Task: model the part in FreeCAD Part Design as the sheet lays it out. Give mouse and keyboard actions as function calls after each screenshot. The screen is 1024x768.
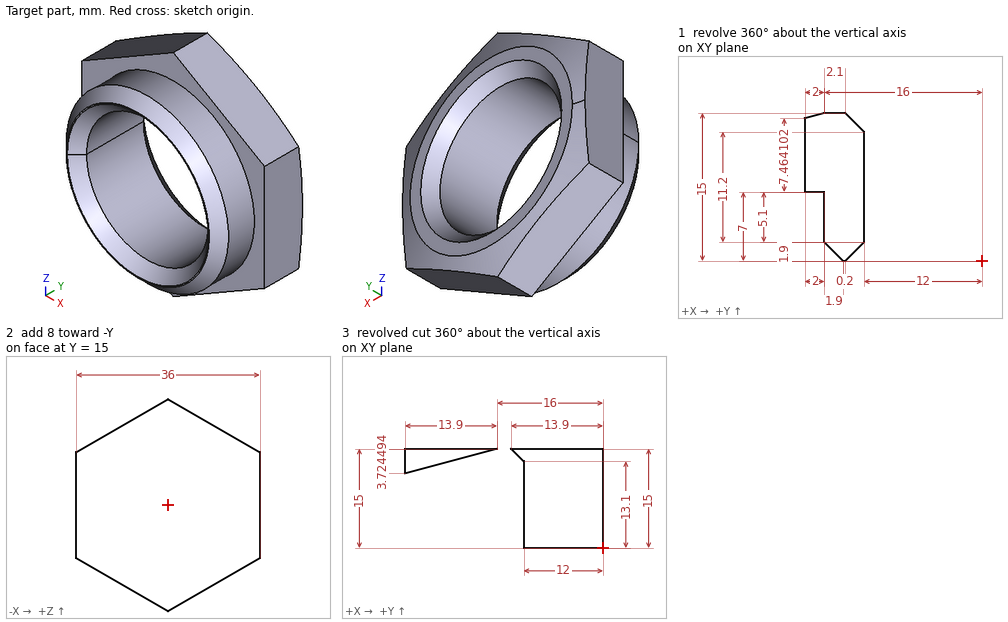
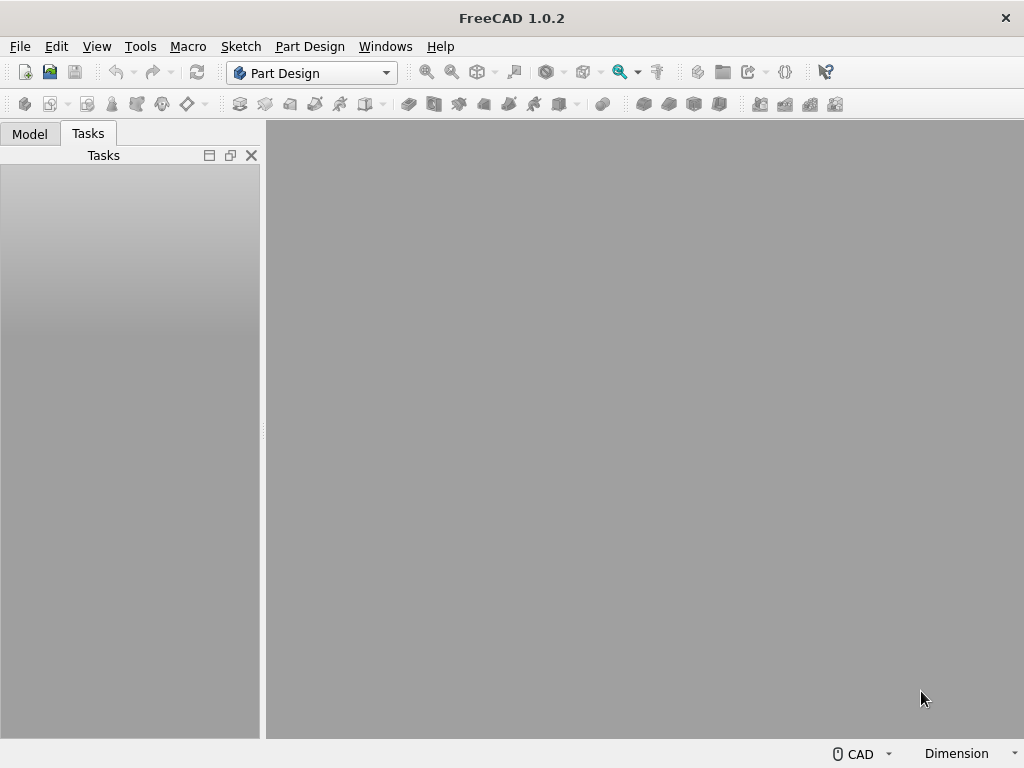
click(25, 72)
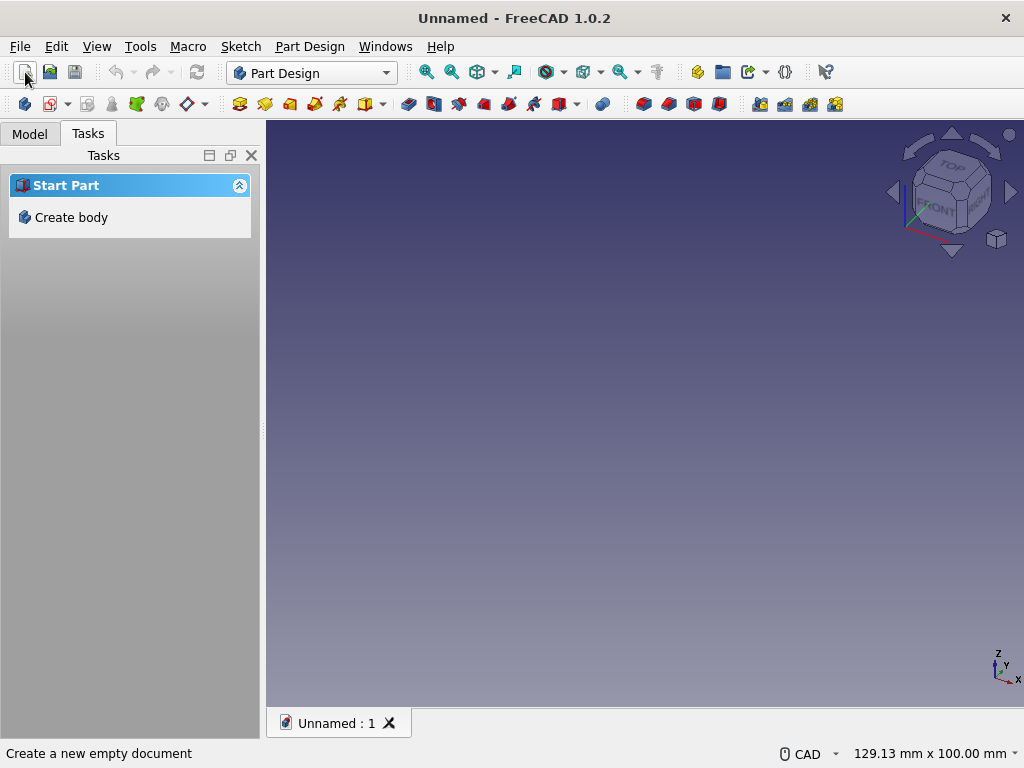
click(50, 104)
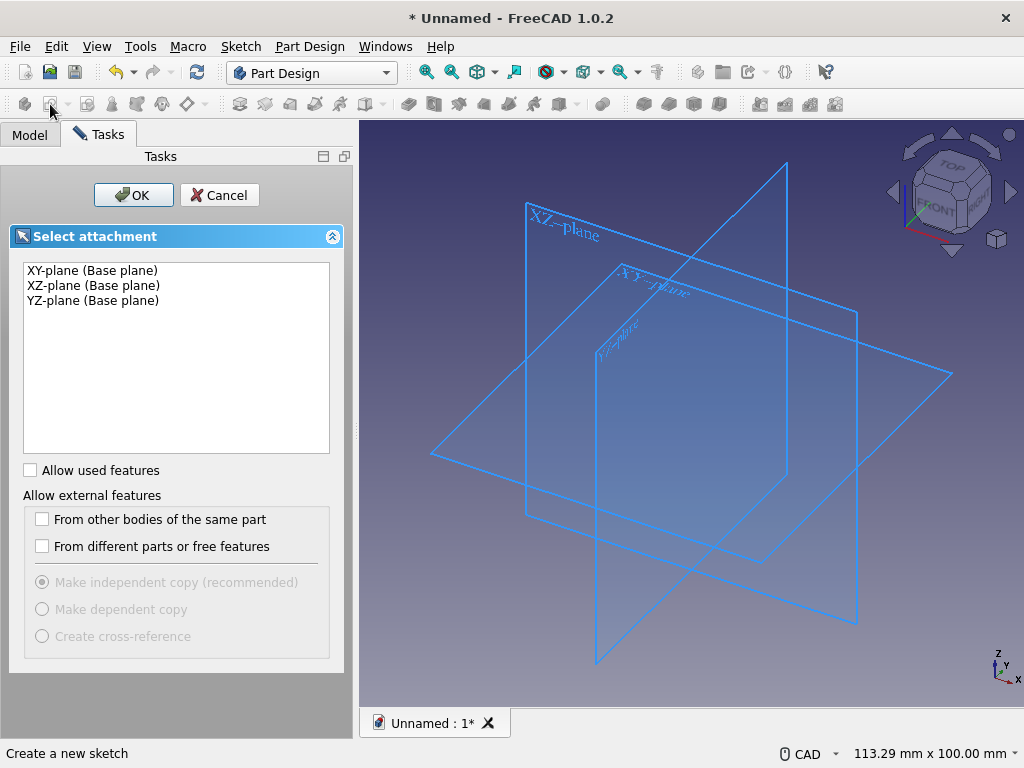
click(84, 270)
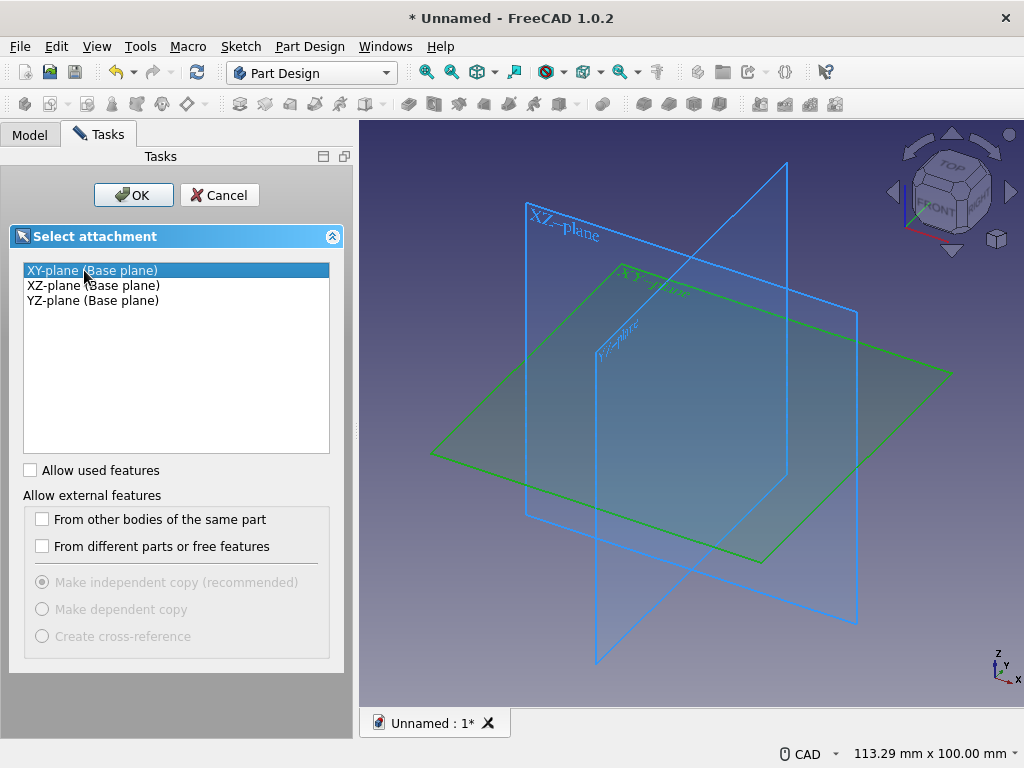
click(134, 195)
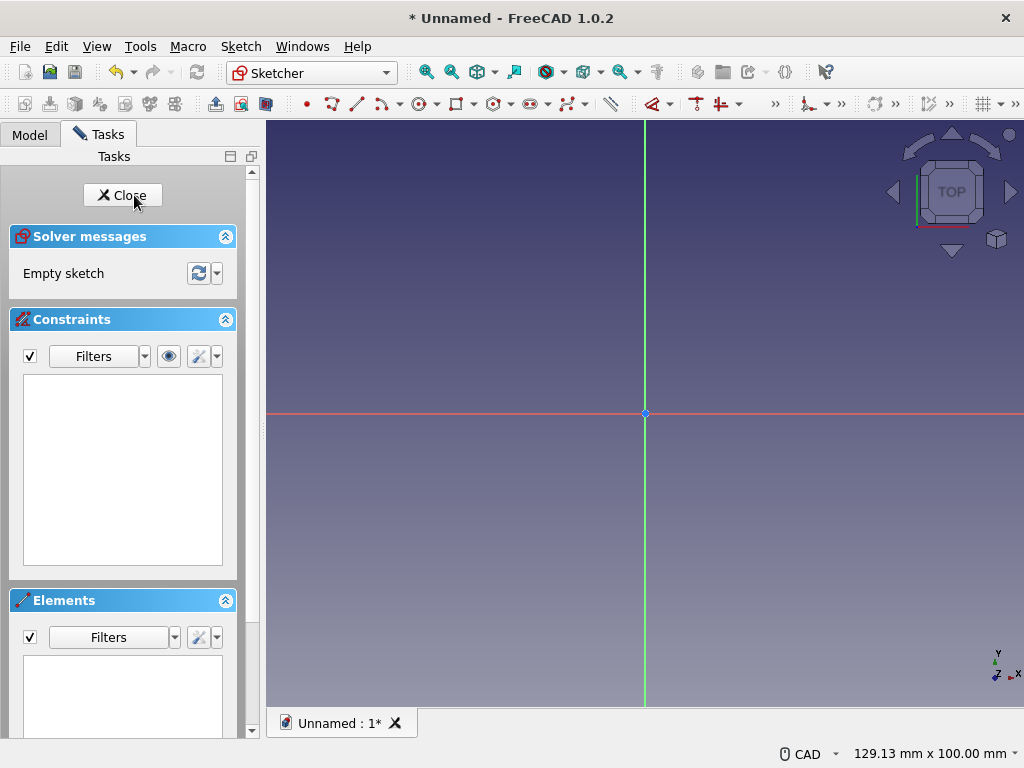
scroll(597, 355, up, 7)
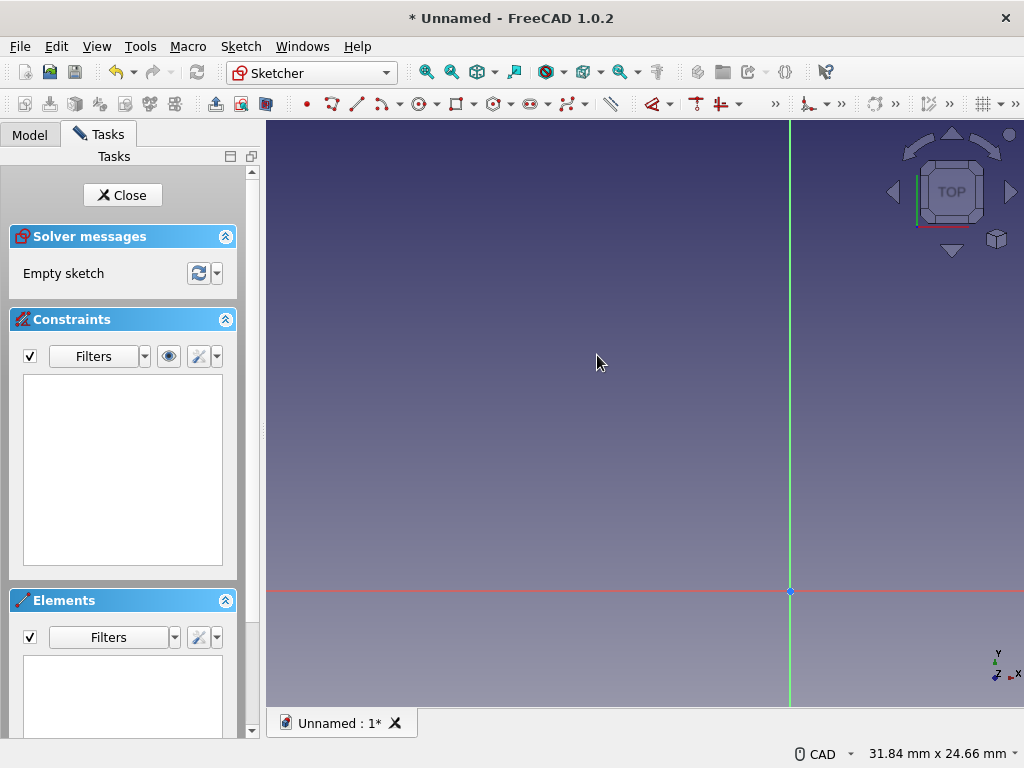
key(g)
key(m)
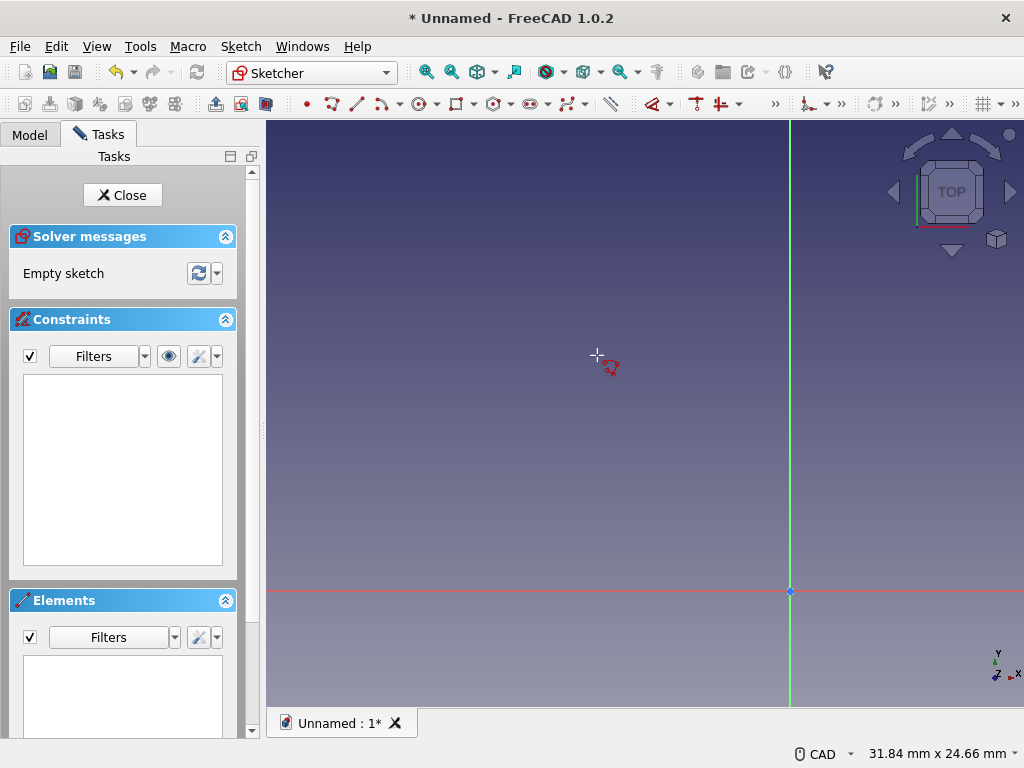
click(505, 546)
click(505, 279)
click(459, 234)
click(409, 234)
click(362, 247)
click(362, 424)
click(409, 424)
click(409, 546)
click(455, 591)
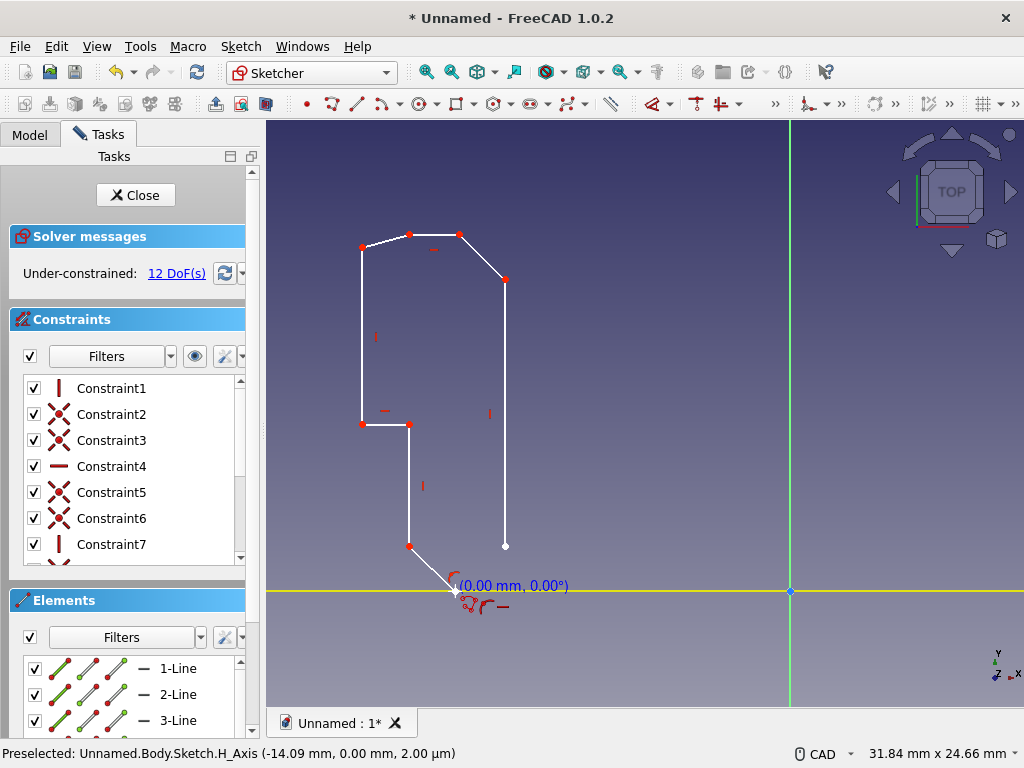
scroll(459, 591, up, 7)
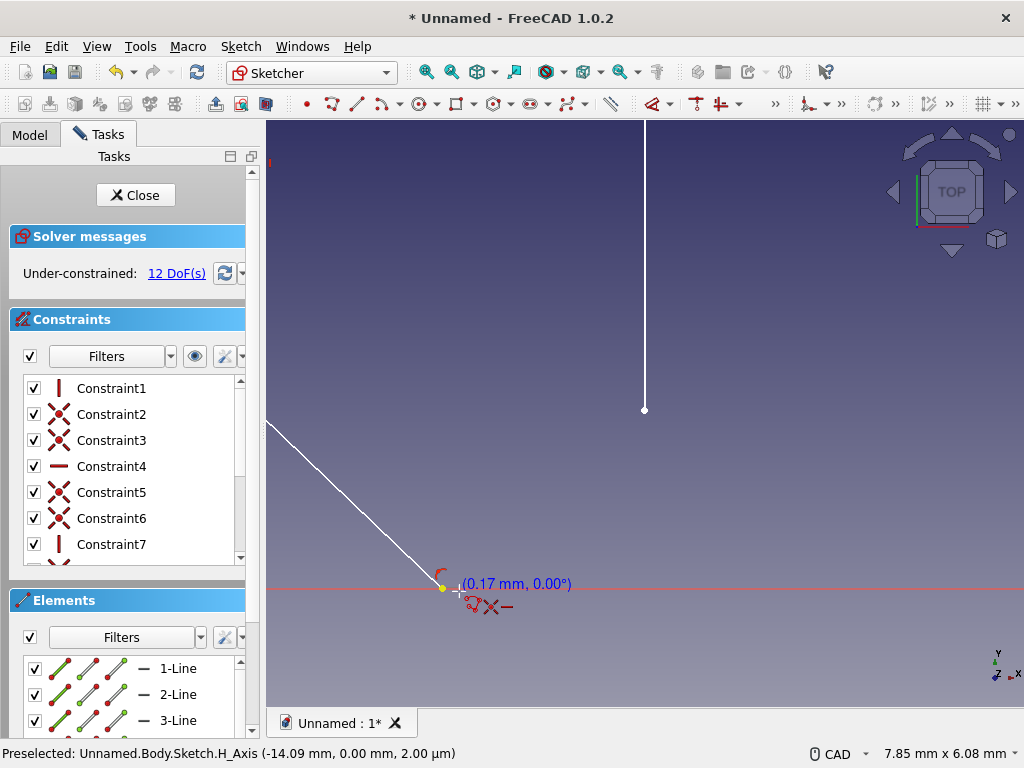
click(460, 580)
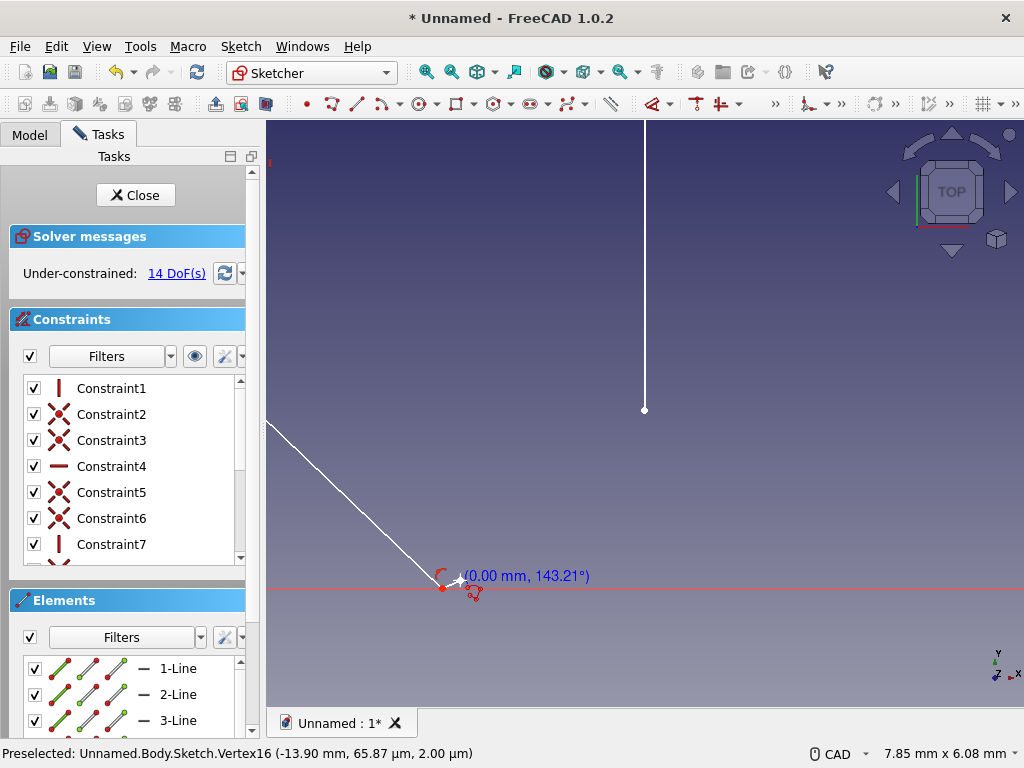
scroll(460, 593, down, 7)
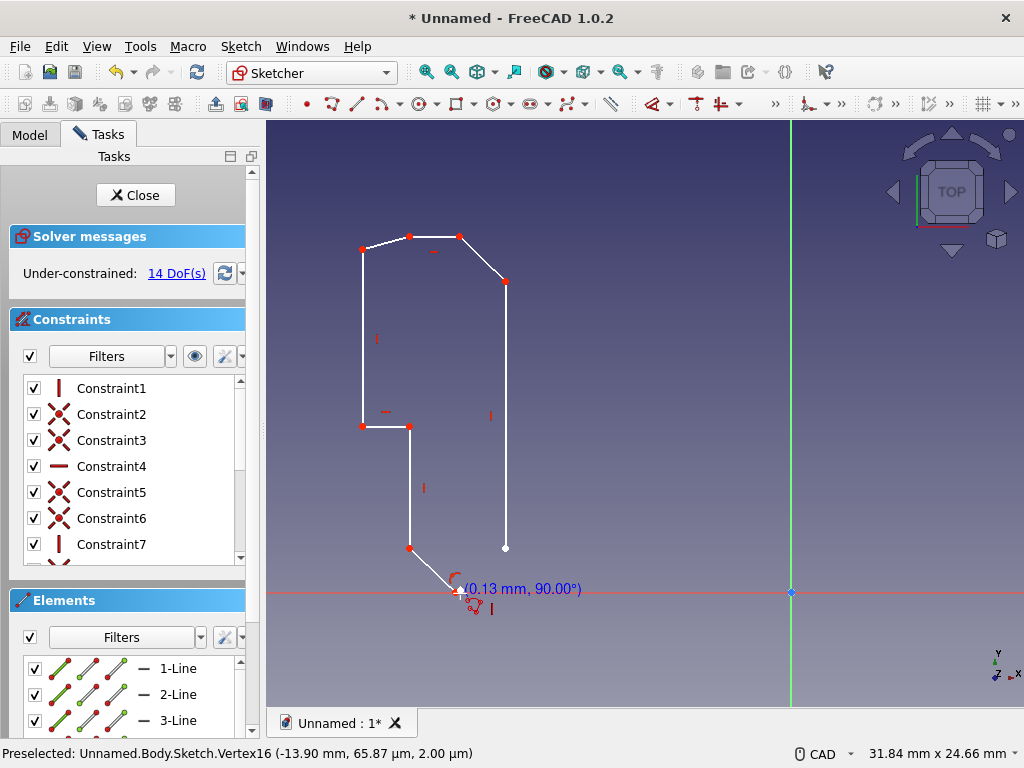
click(506, 549)
key(Escape)
key(Escape)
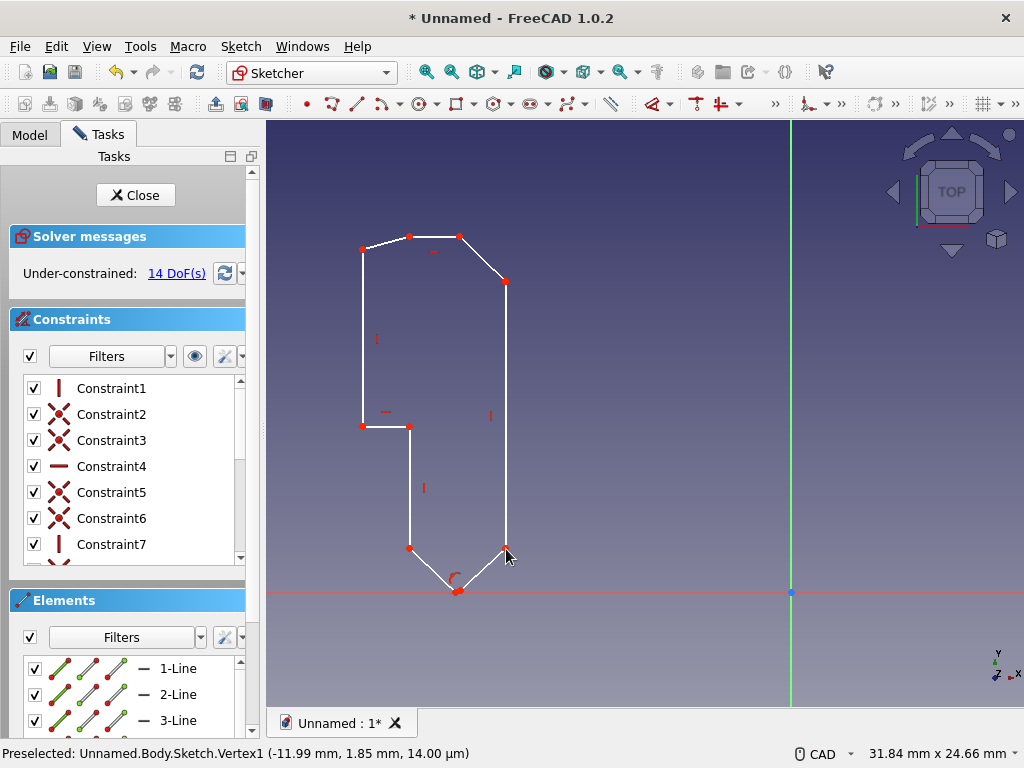
scroll(458, 592, up, 9)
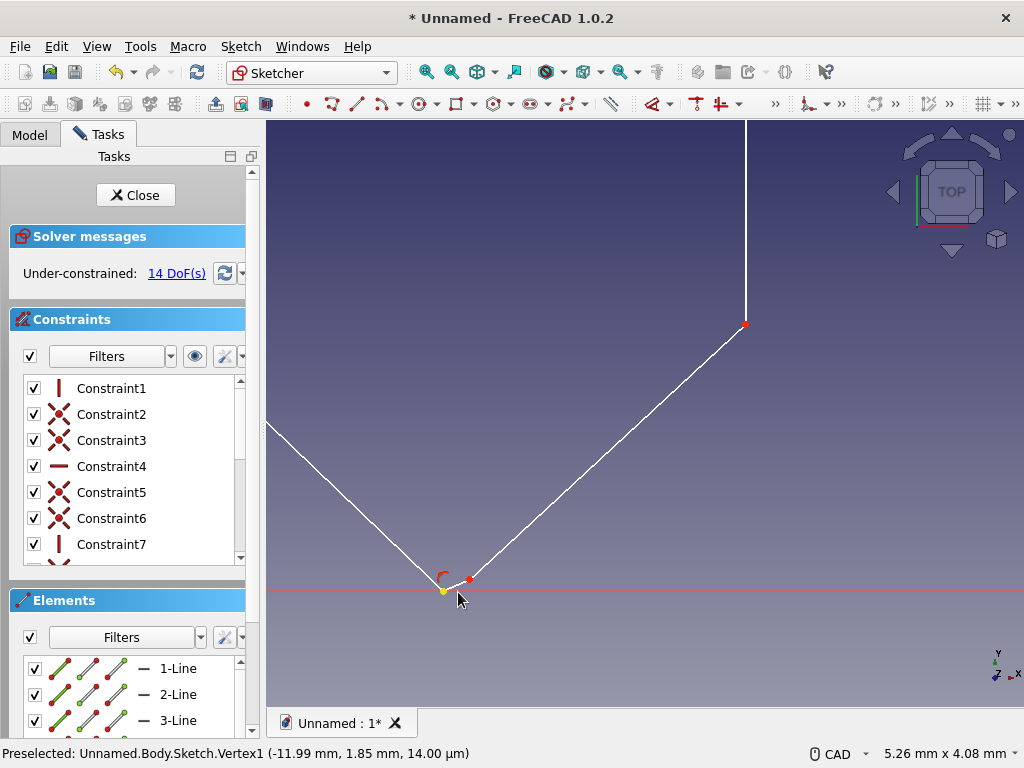
click(457, 585)